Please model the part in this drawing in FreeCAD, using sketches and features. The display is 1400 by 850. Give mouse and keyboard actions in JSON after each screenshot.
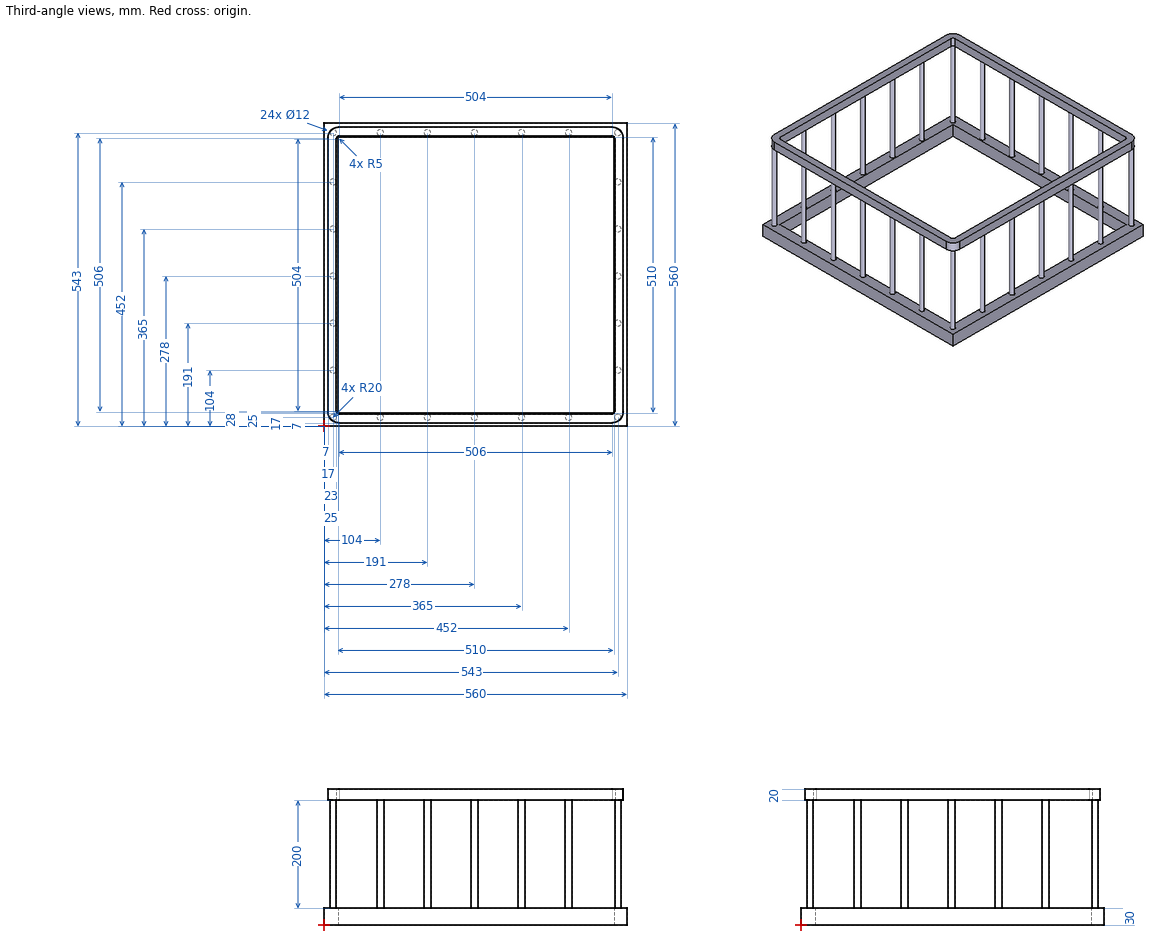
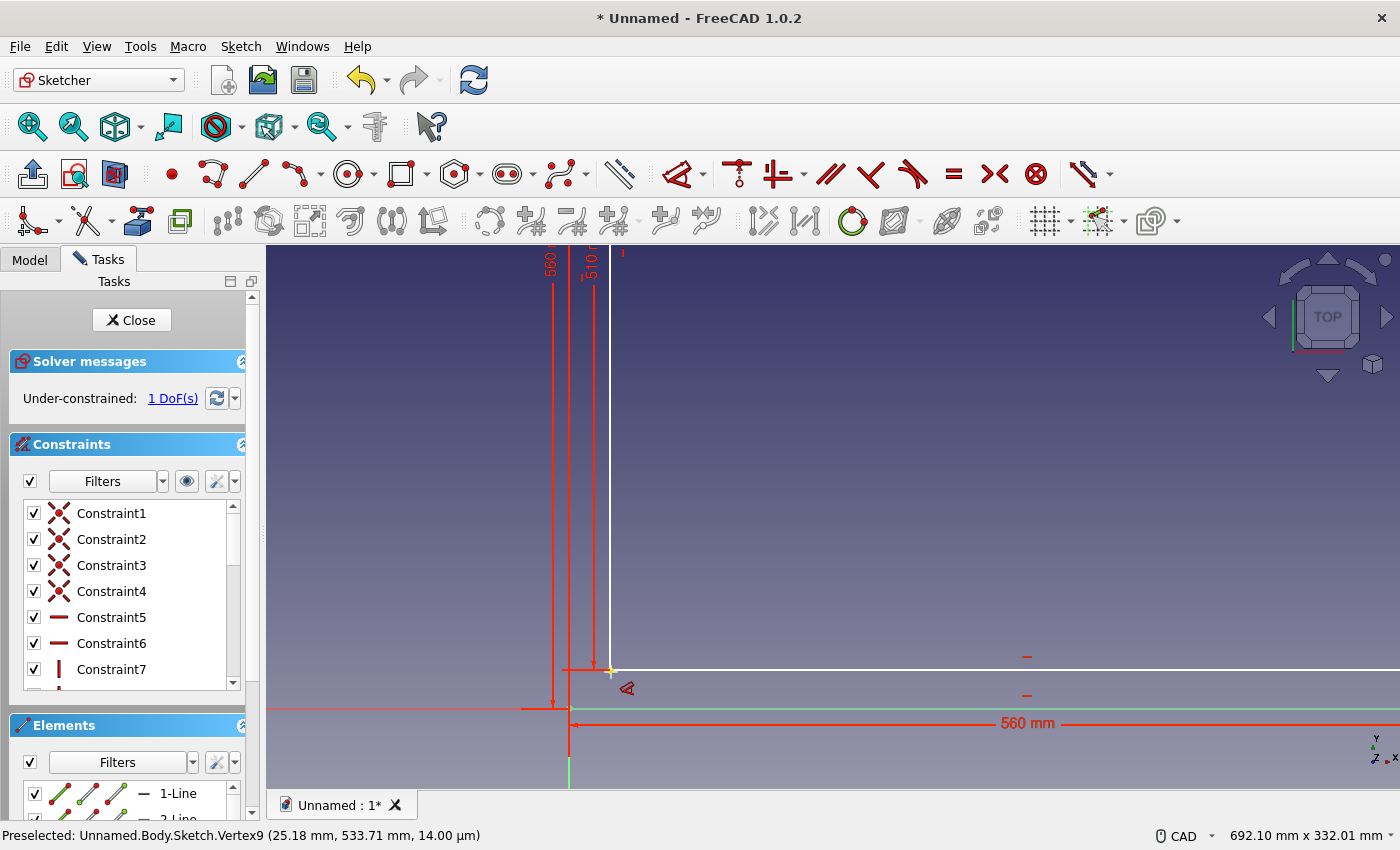
{"action": "left_click", "coordinate": [610, 670]}
{"action": "left_click", "coordinate": [535, 689]}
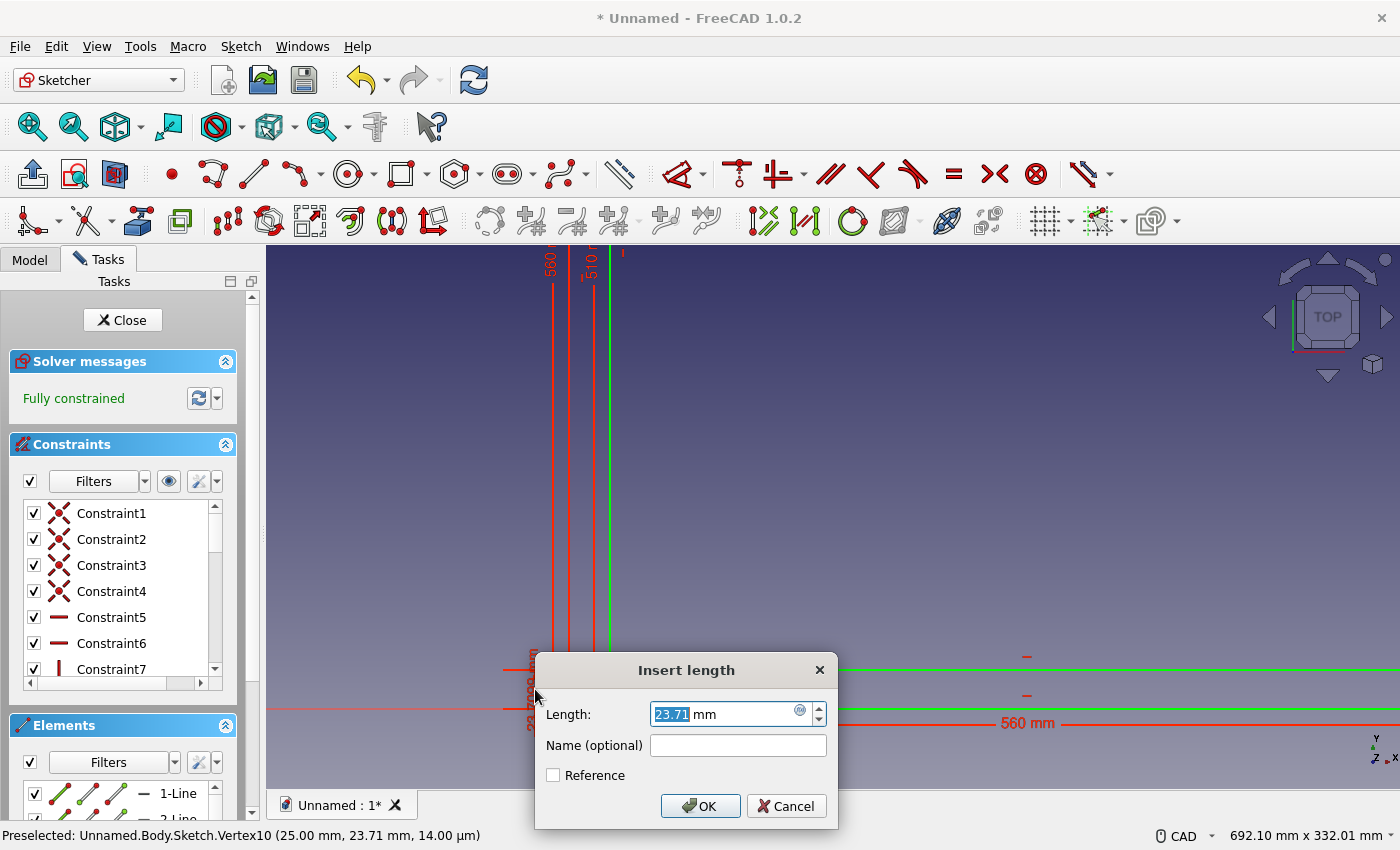
{"action": "type", "text": "25"}
{"action": "key", "text": "Return"}
{"action": "key", "text": "Escape"}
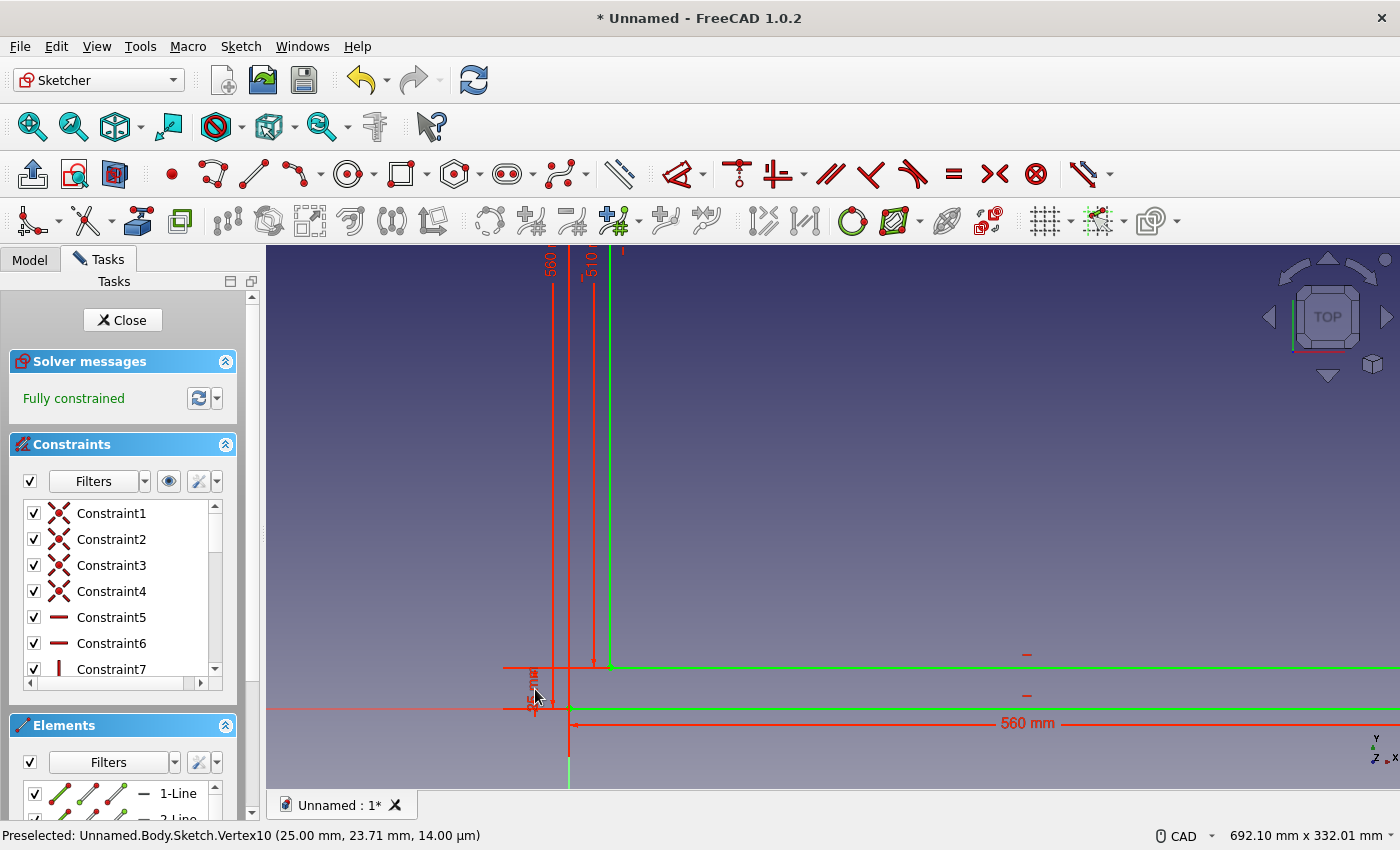
{"action": "left_click", "coordinate": [123, 320]}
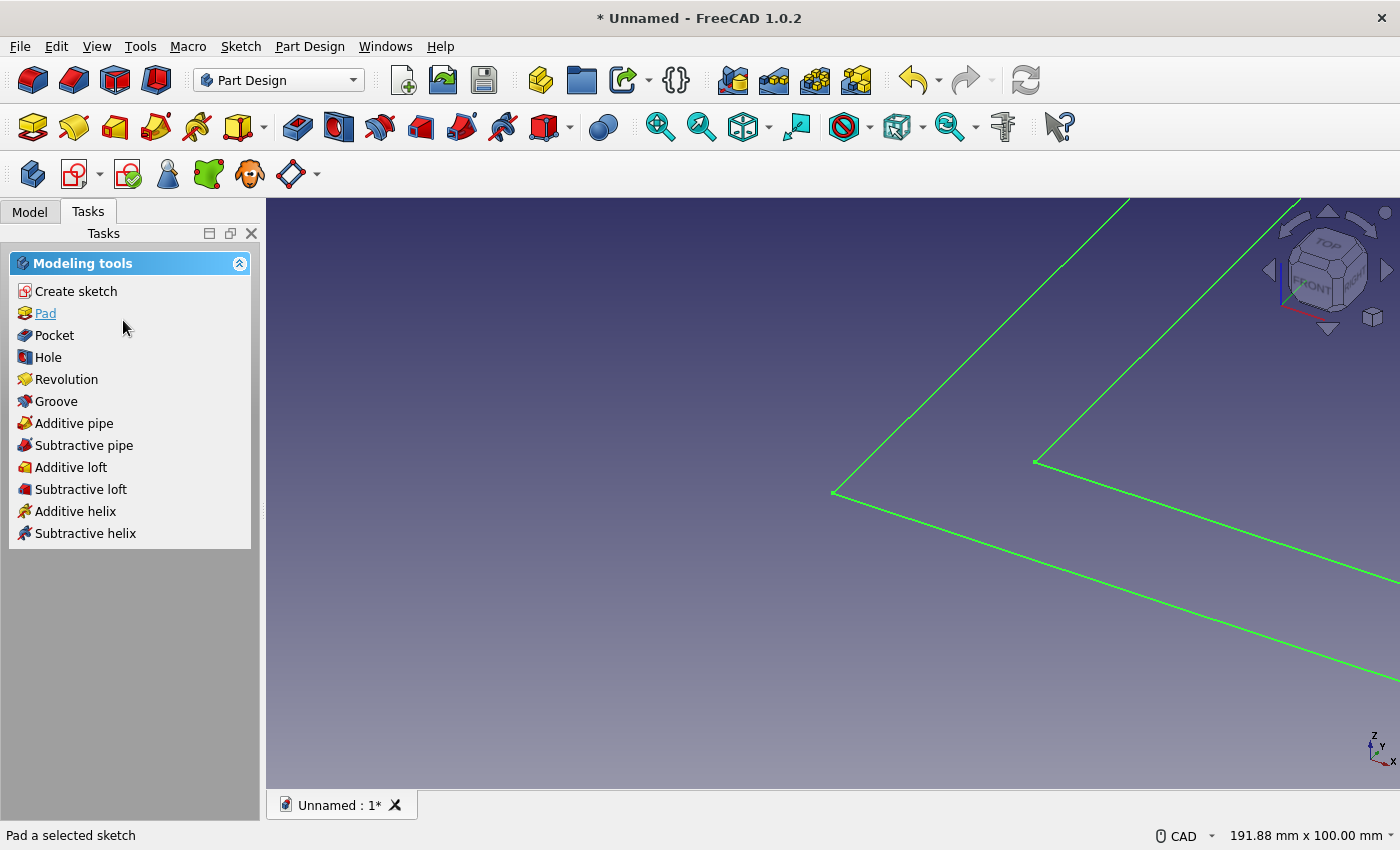
{"action": "left_click", "coordinate": [33, 128]}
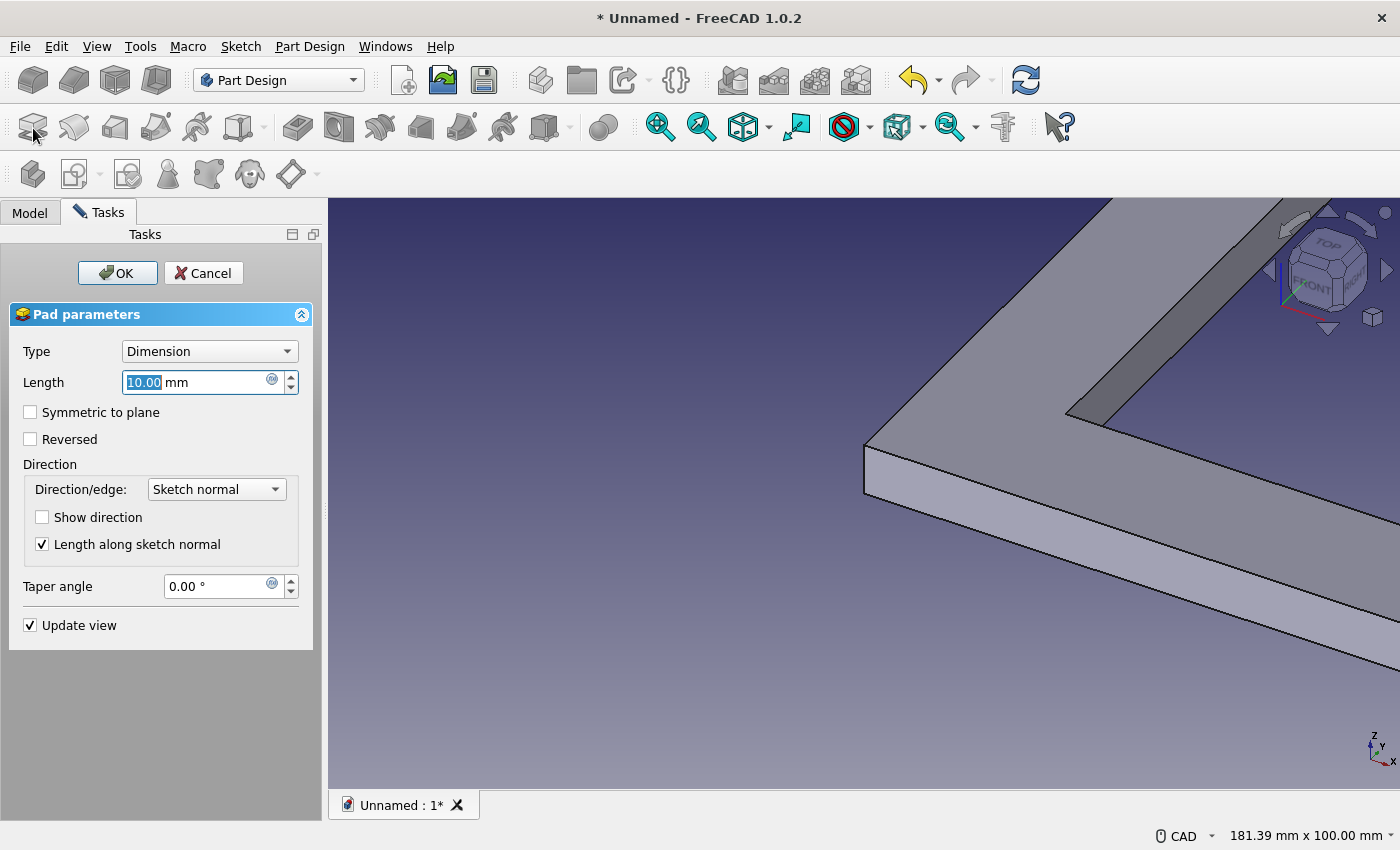
{"action": "type", "text": "30"}
{"action": "key", "text": "Tab"}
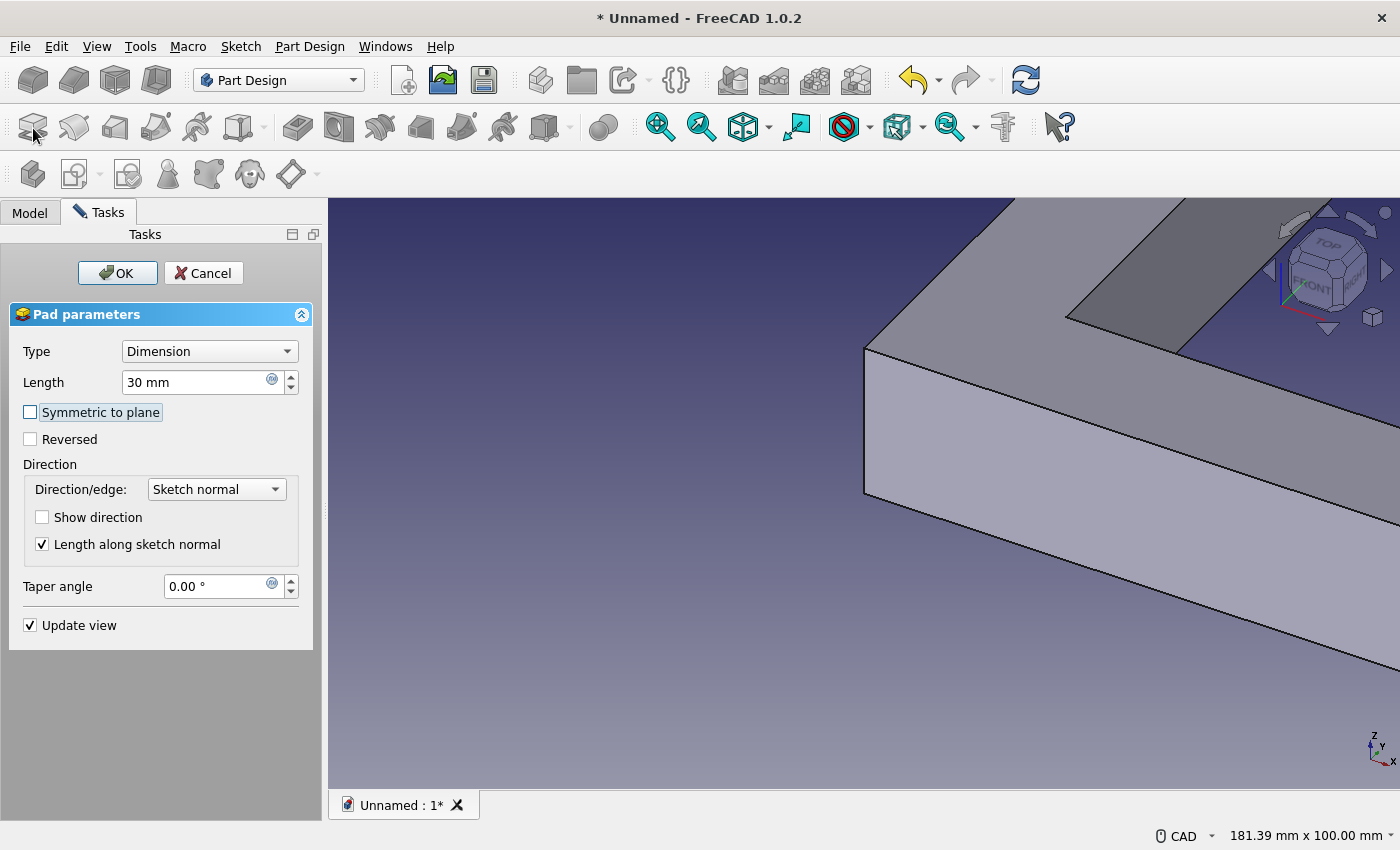
{"action": "left_click", "coordinate": [118, 273]}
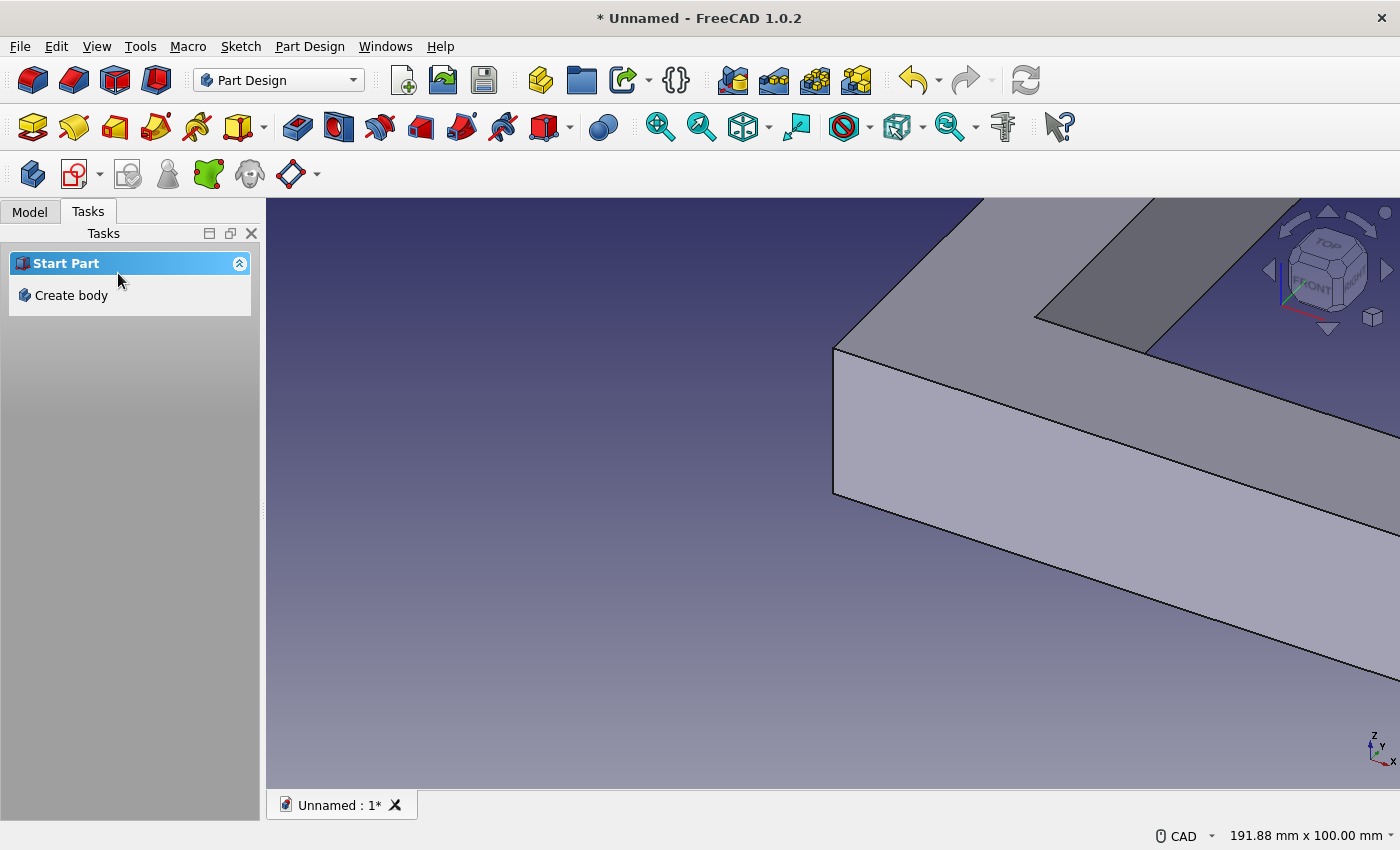
{"action": "left_click", "coordinate": [661, 128]}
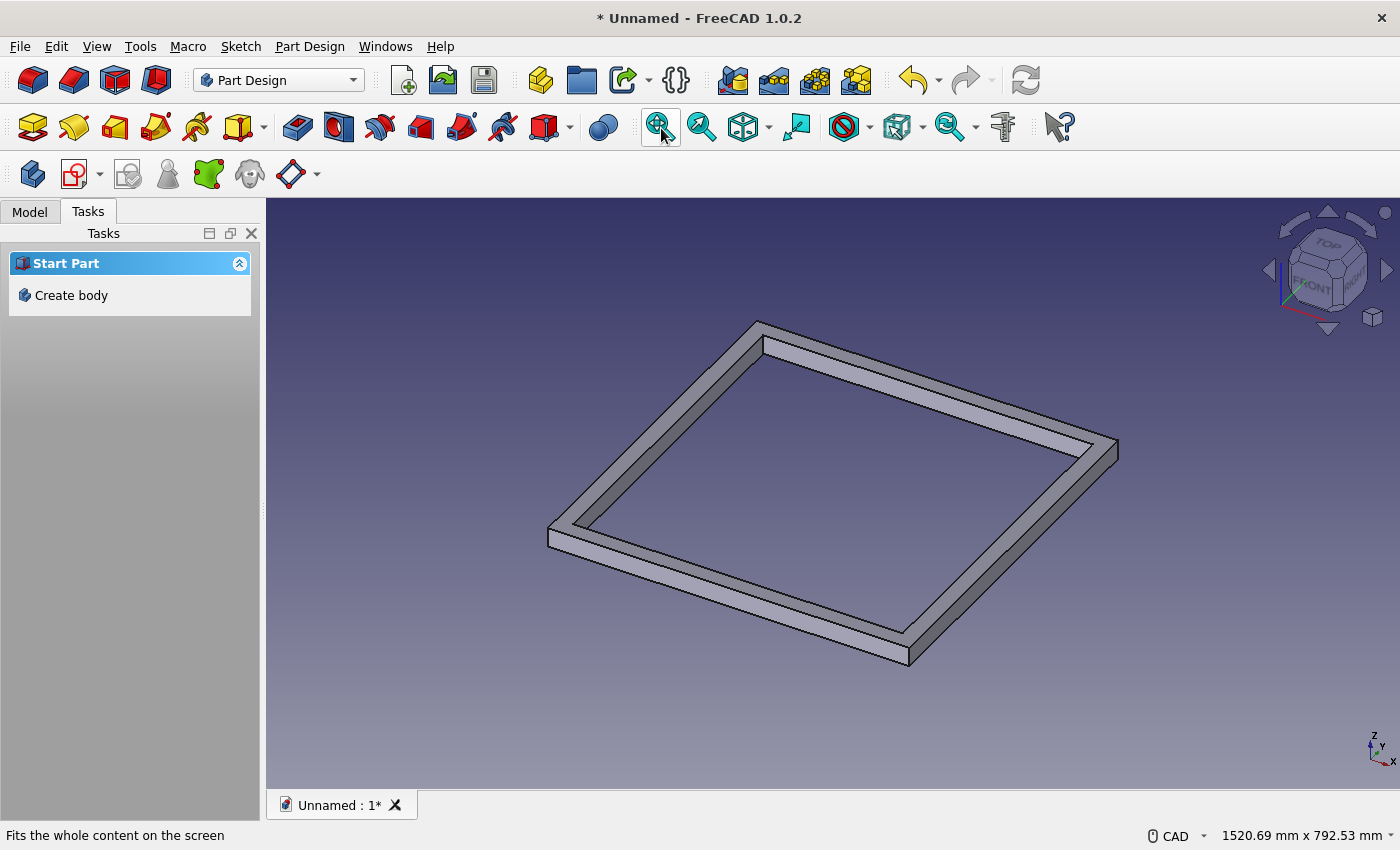
{"action": "left_click", "coordinate": [1038, 505]}